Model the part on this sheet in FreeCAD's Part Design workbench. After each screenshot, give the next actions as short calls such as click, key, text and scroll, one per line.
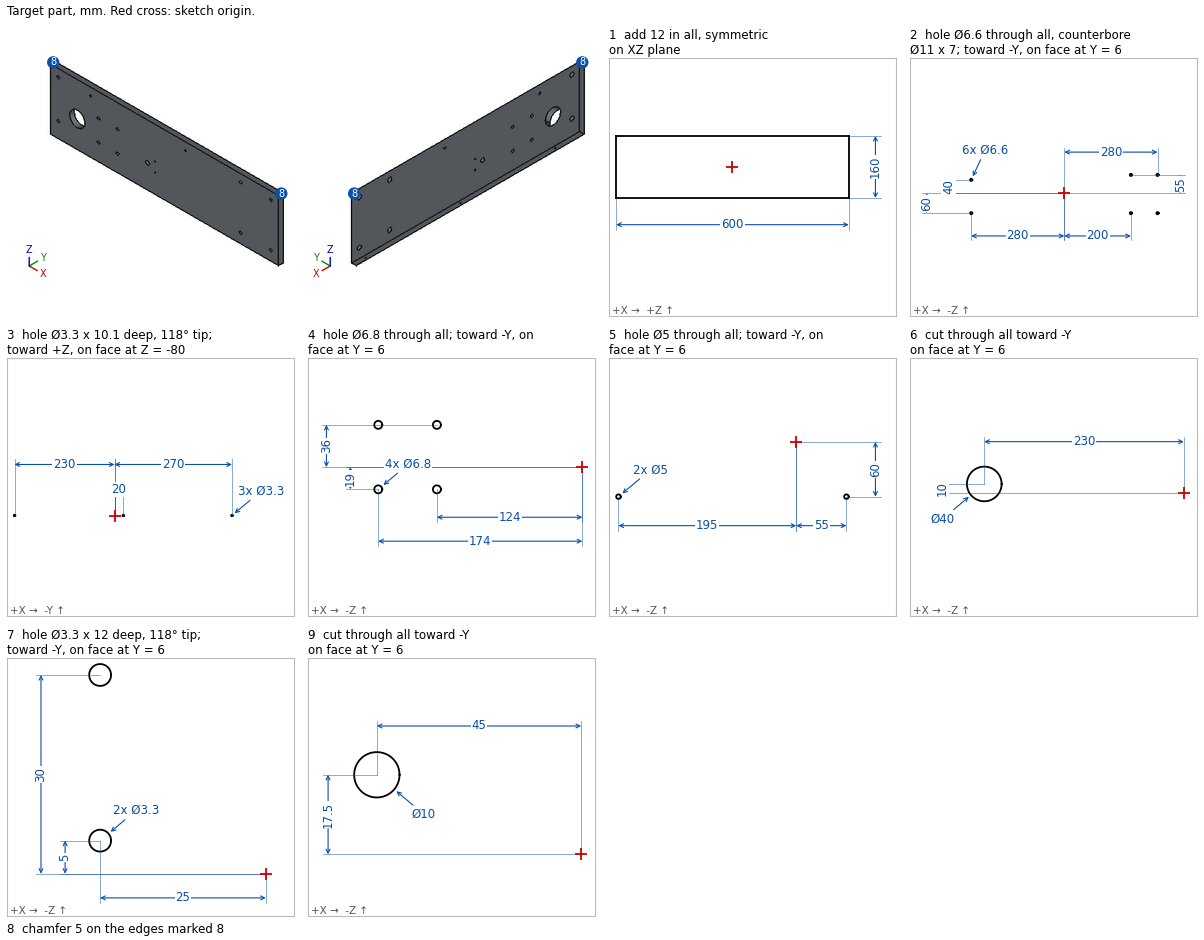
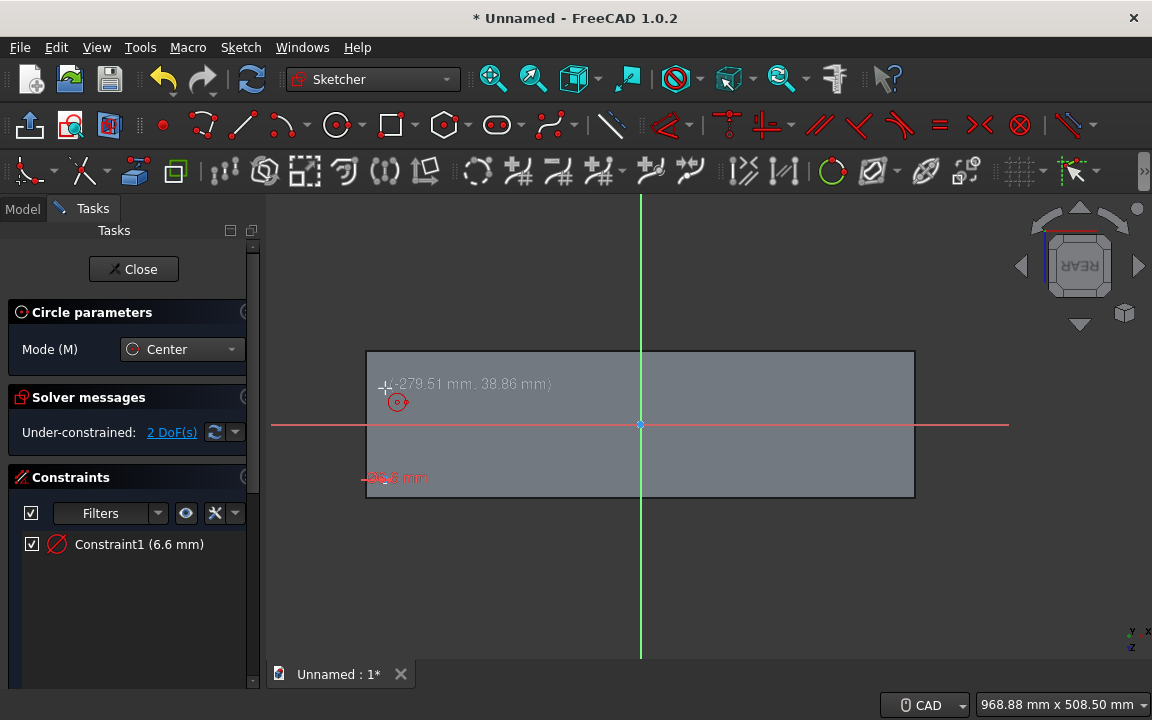
click(385, 388)
move(387, 386)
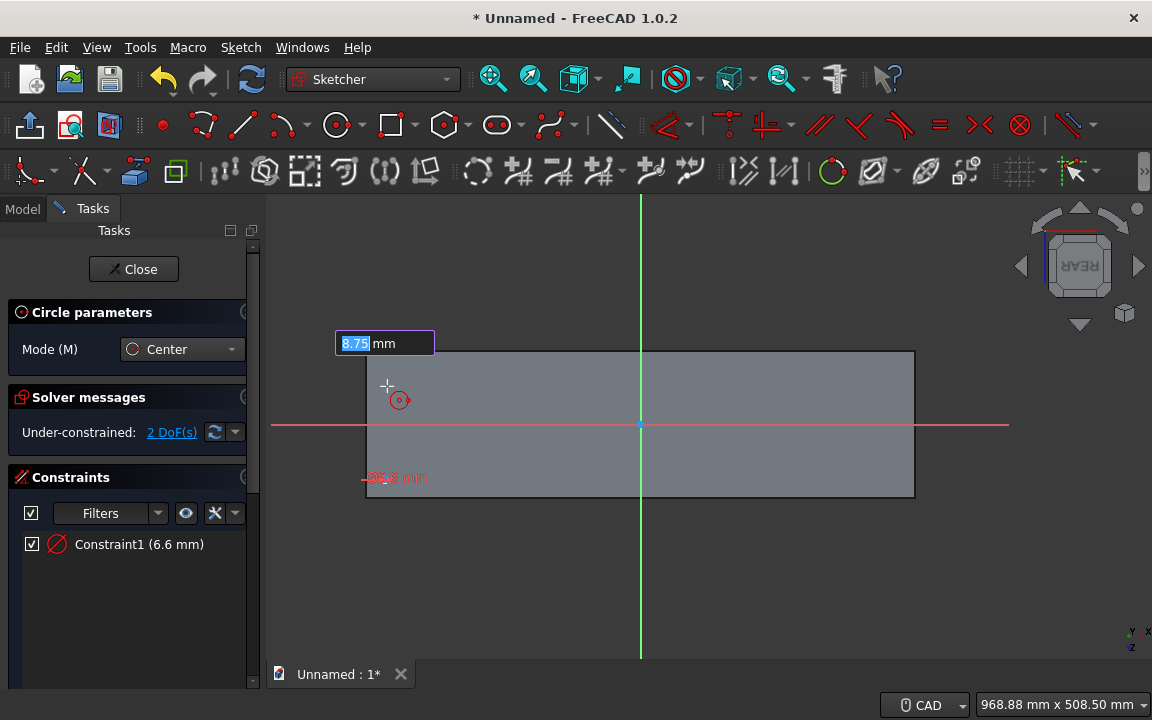
text(6.6)
key(Return)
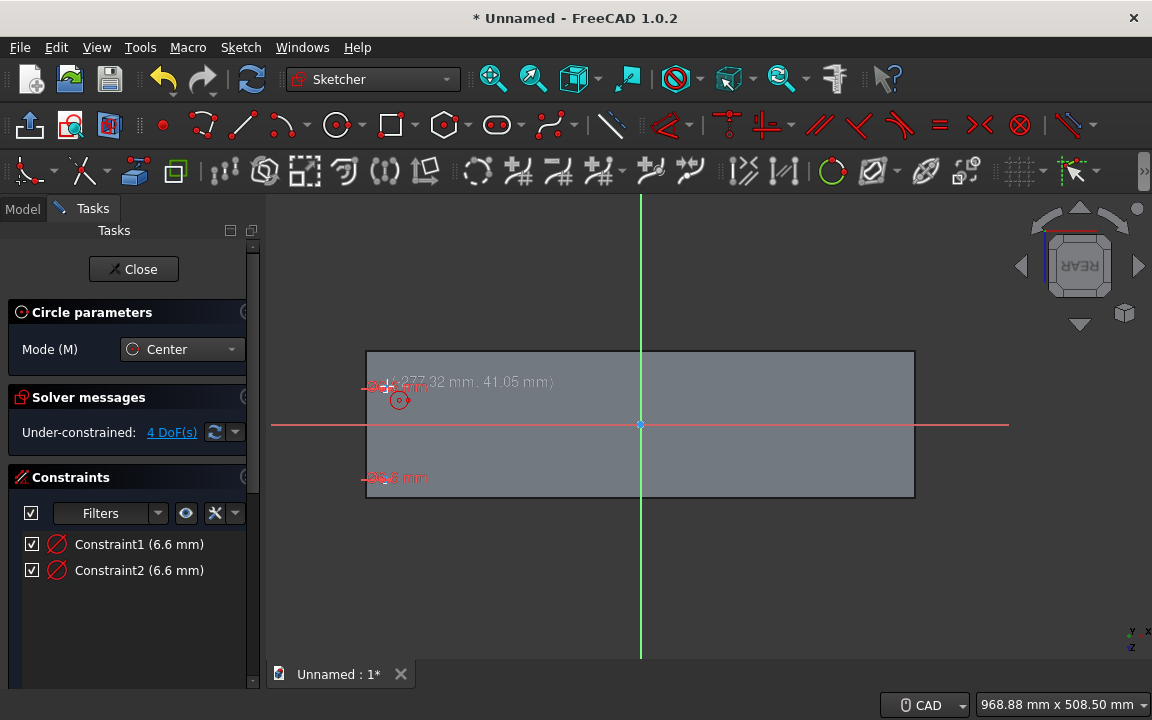
scroll(823, 479, up, 11)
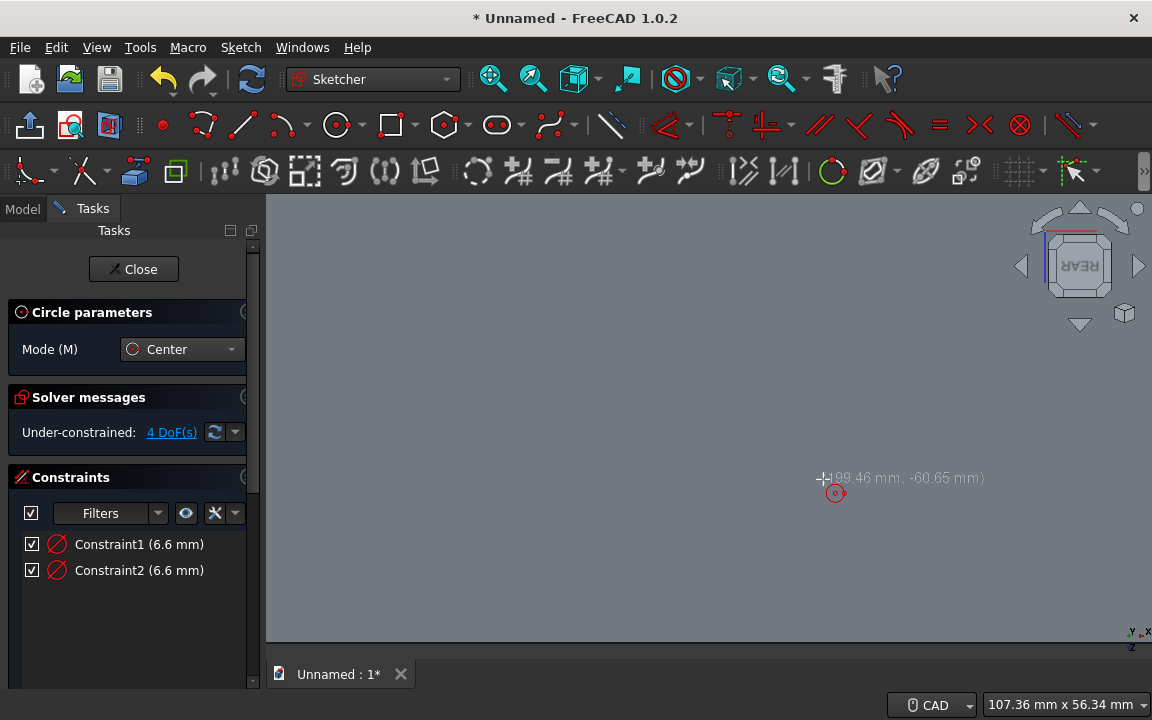
scroll(824, 479, down, 11)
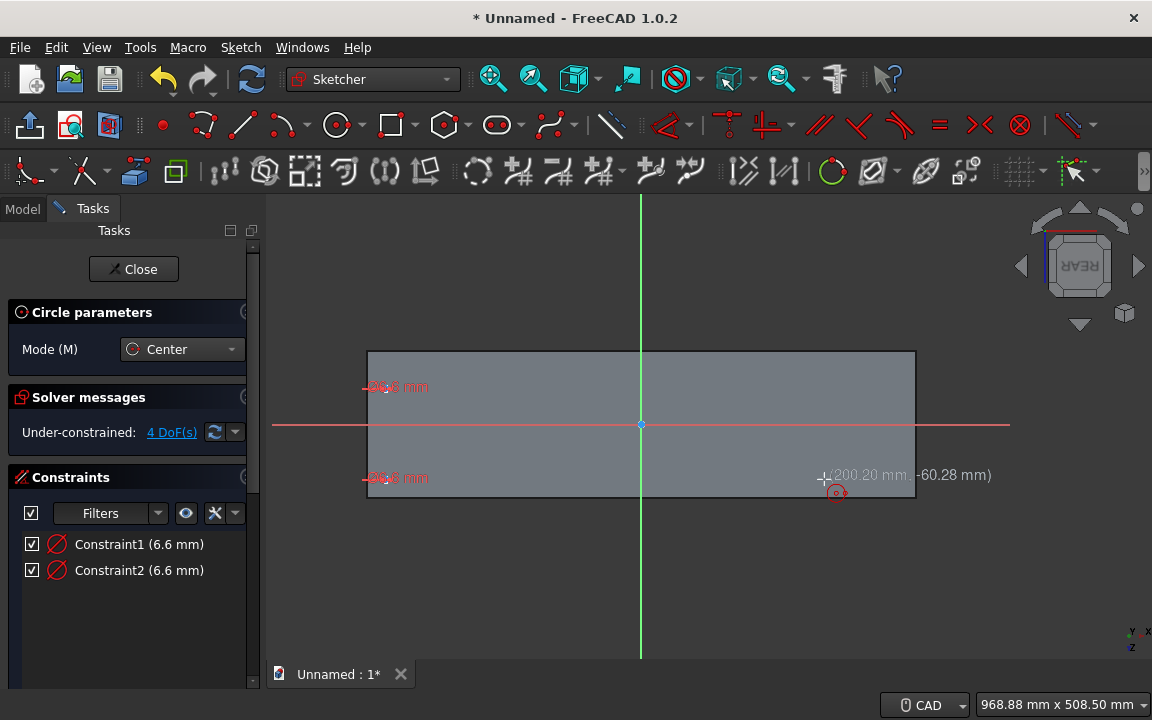
click(824, 479)
move(827, 477)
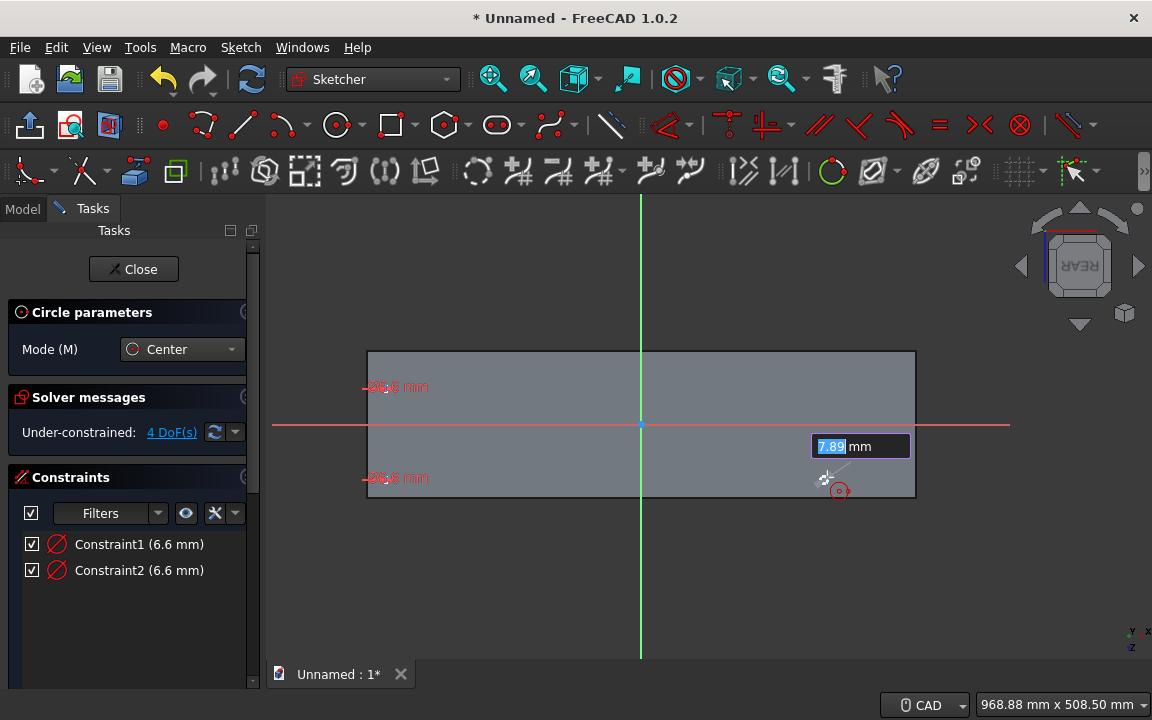
text(6.6)
key(Return)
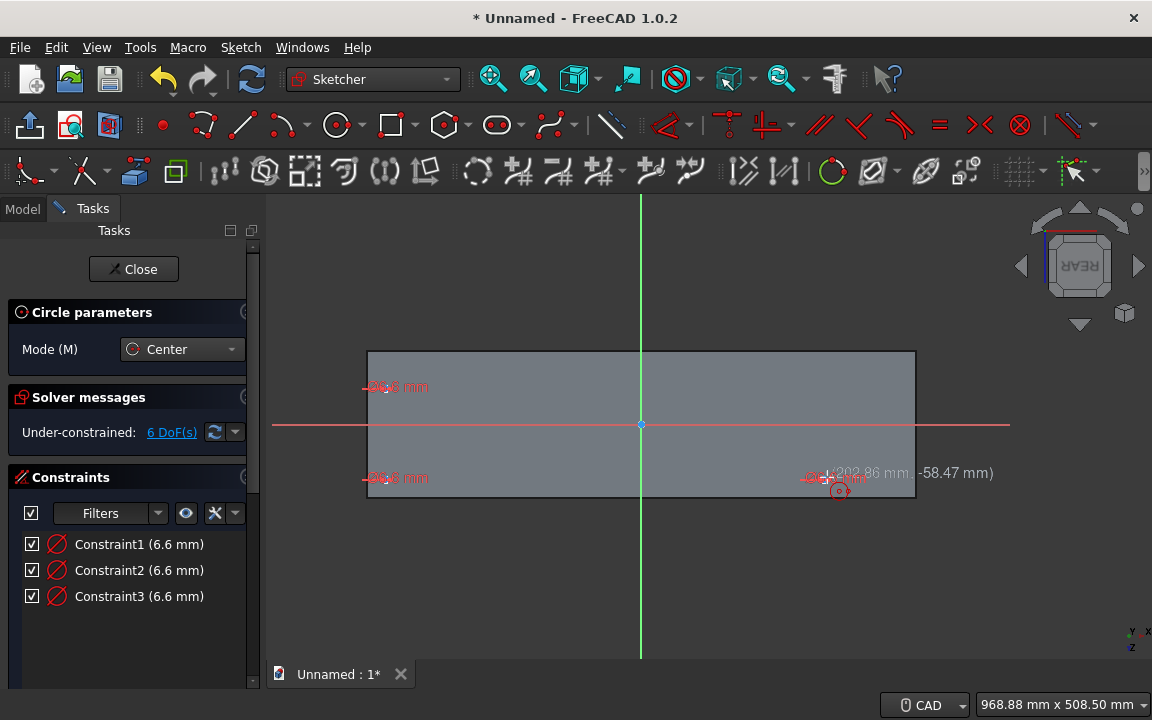
scroll(824, 374, up, 11)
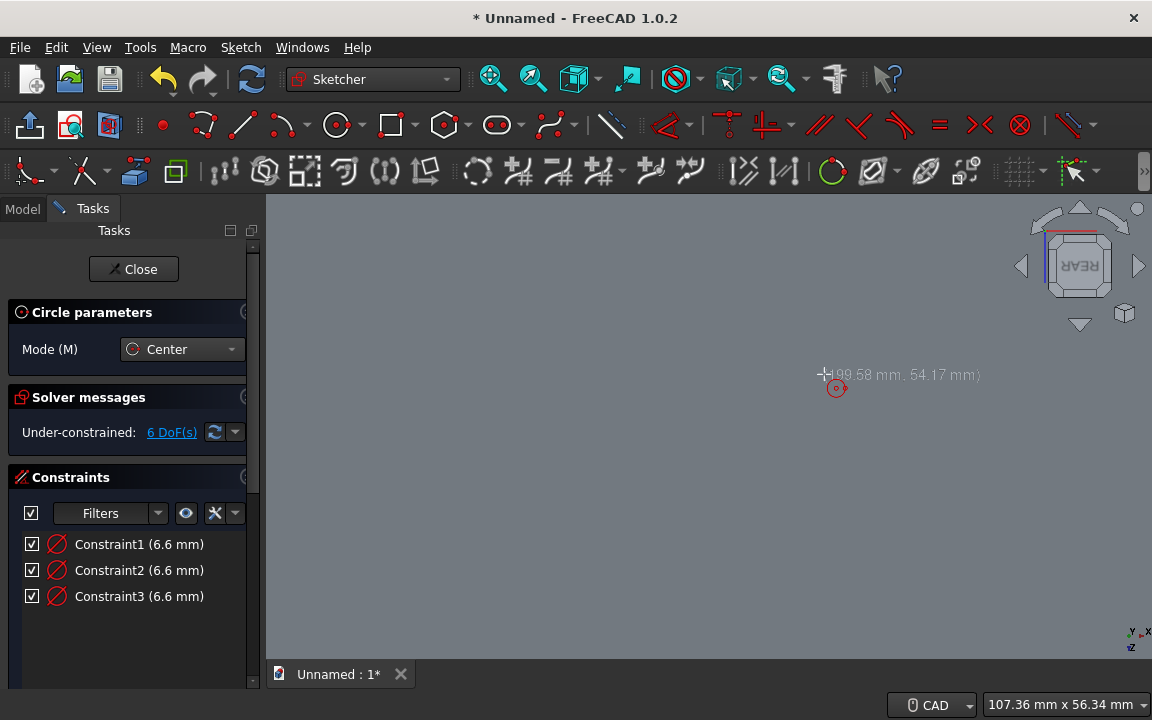
scroll(824, 374, down, 11)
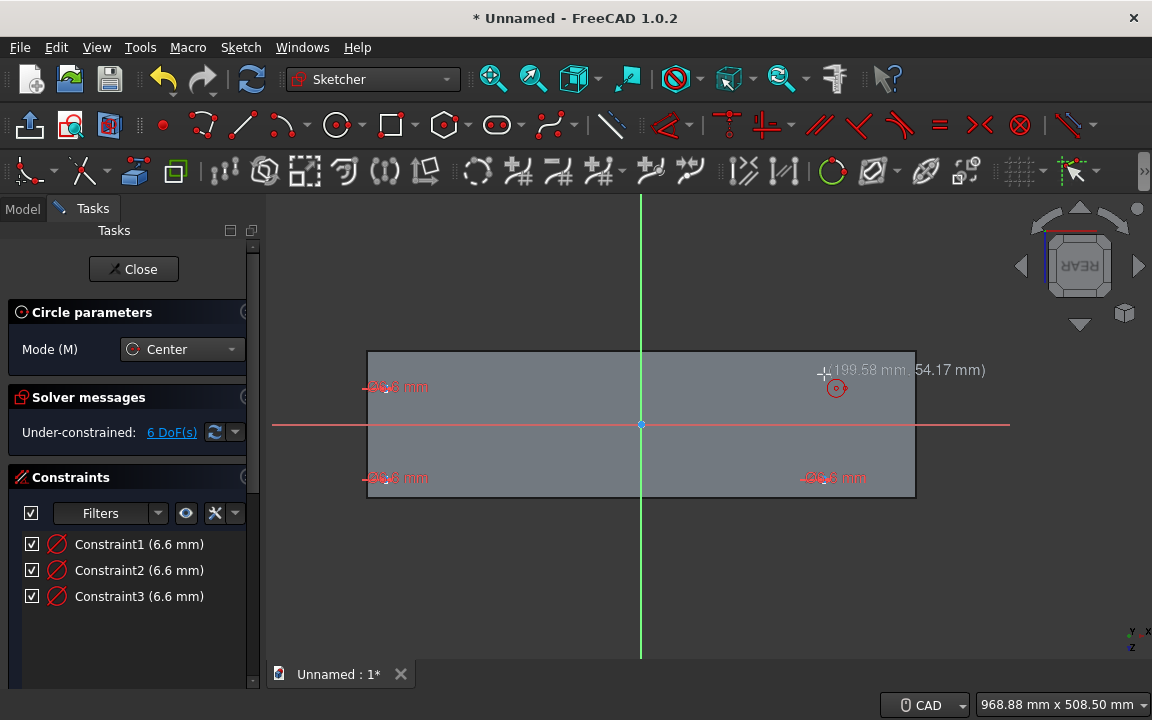
click(824, 374)
move(827, 372)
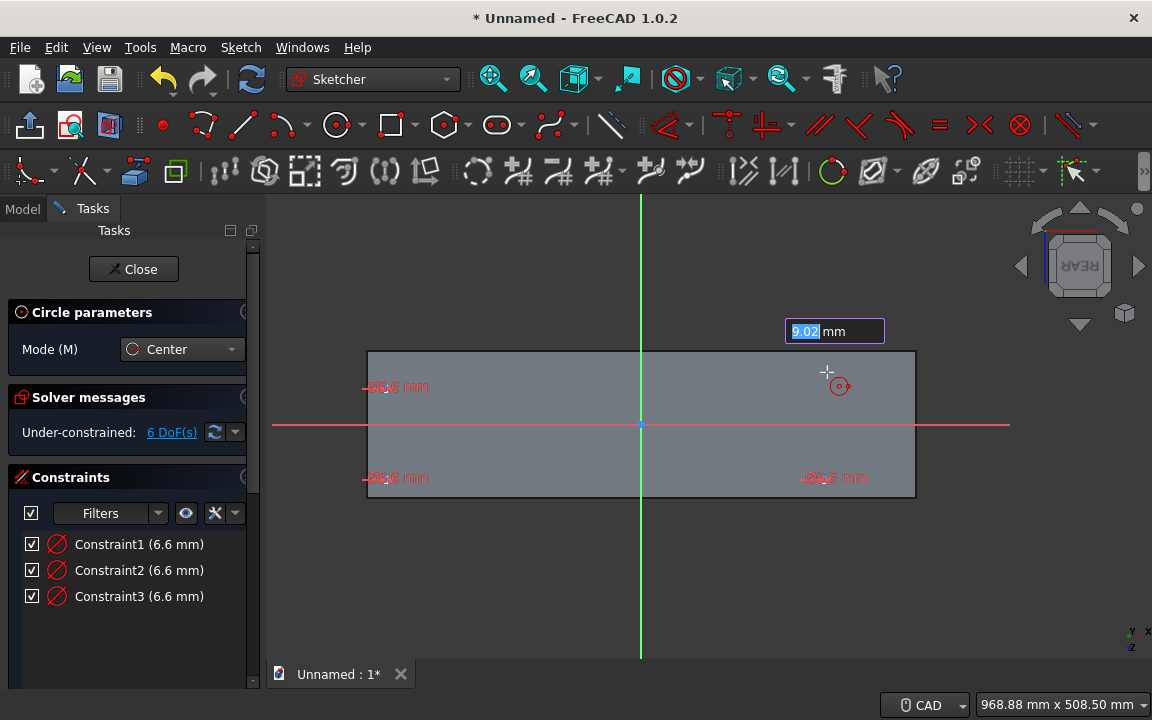
text(6.6)
key(Return)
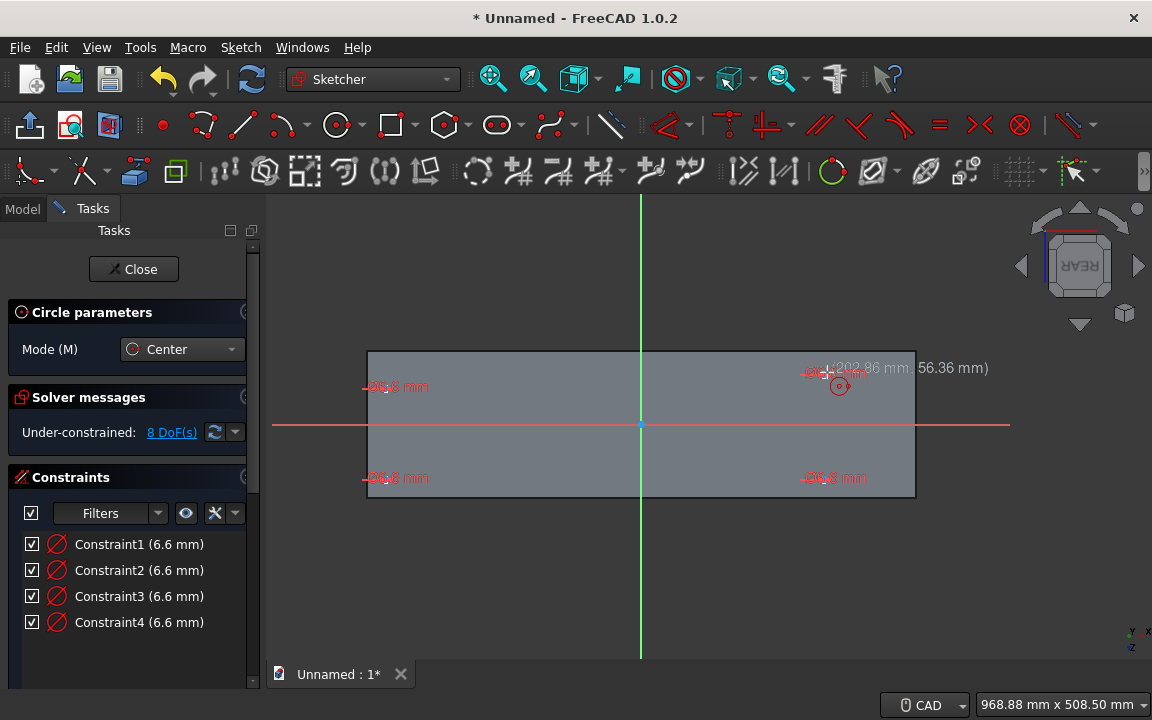
scroll(898, 374, up, 11)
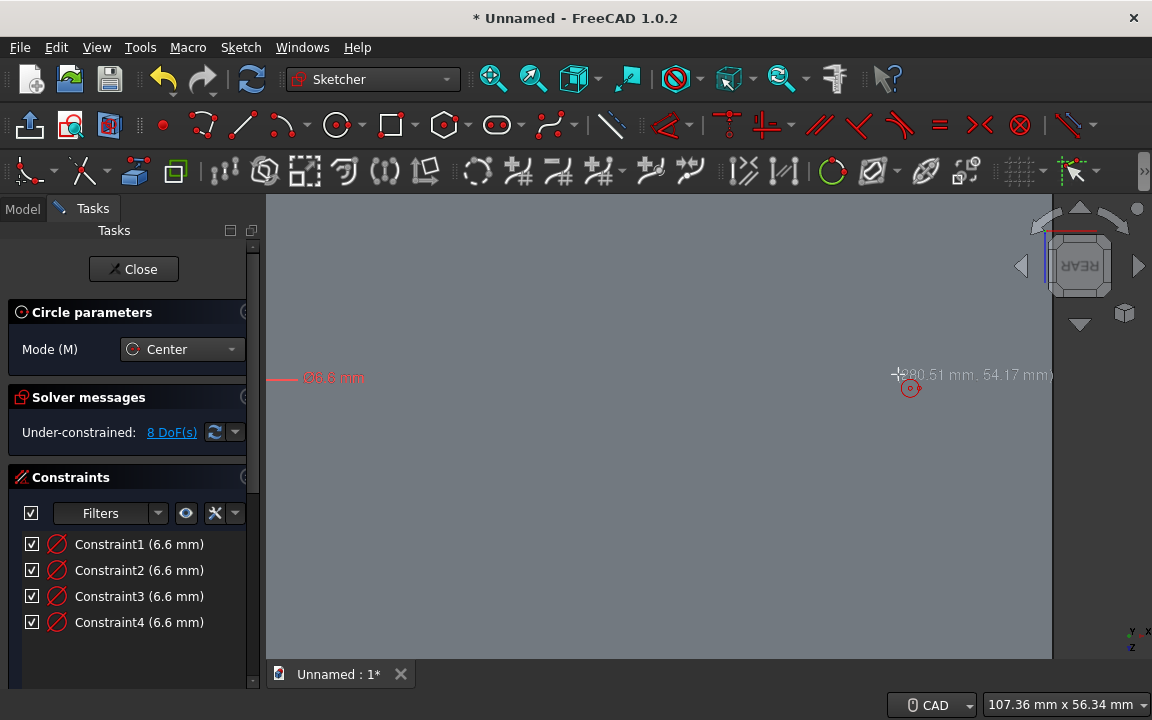
scroll(898, 374, down, 11)